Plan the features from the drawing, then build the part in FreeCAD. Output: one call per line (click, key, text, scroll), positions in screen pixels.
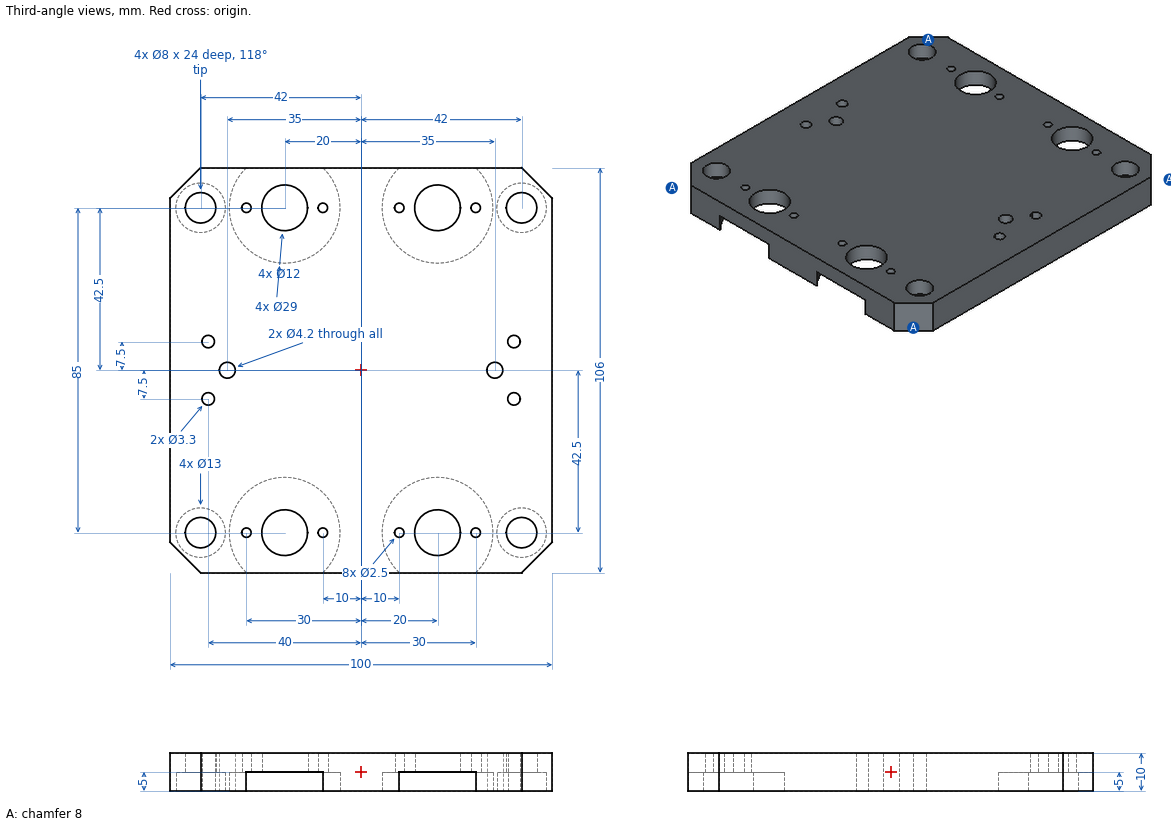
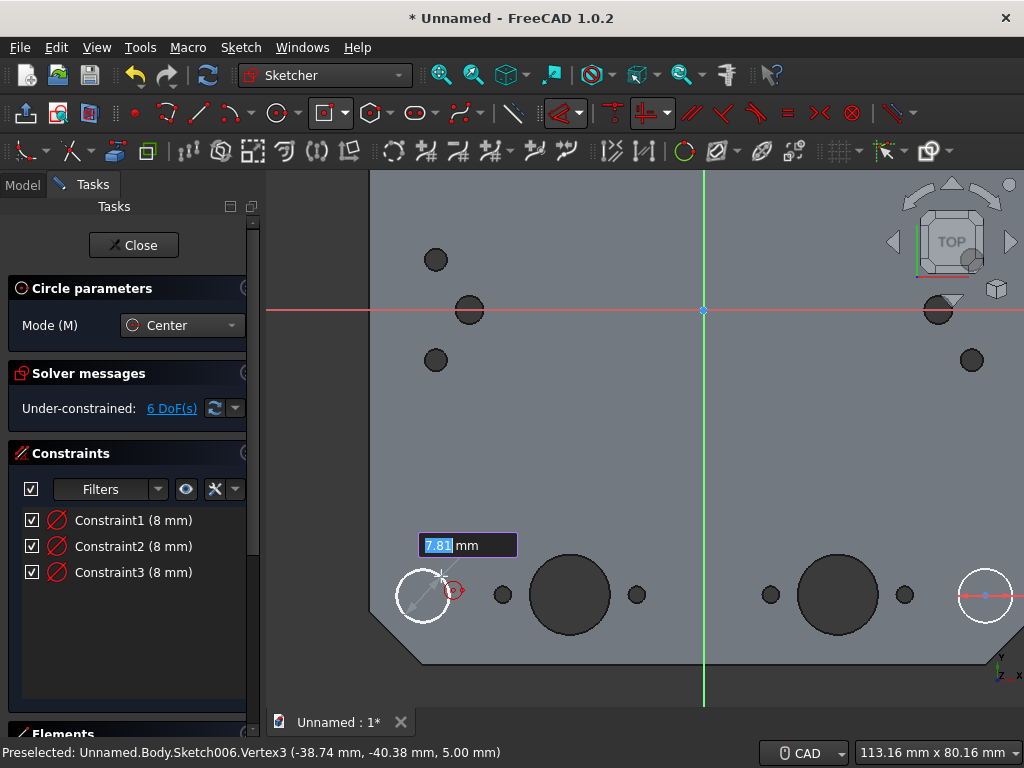
text(8)
key(Return)
key(Escape)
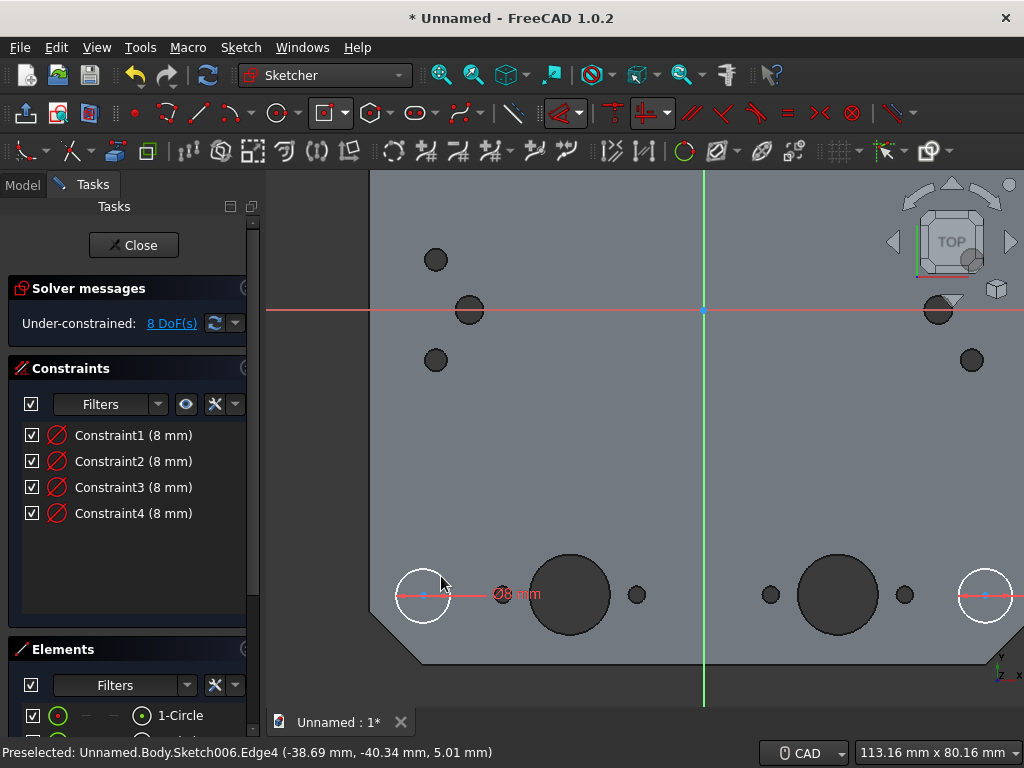
scroll(422, 595, down, 3)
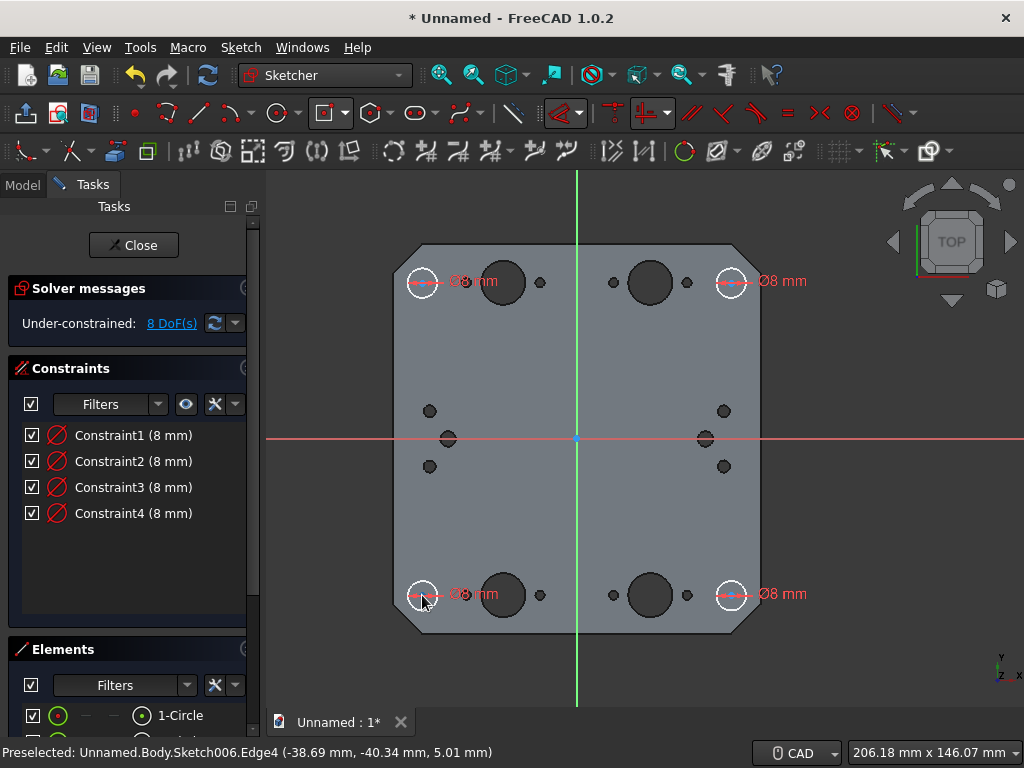
click(422, 283)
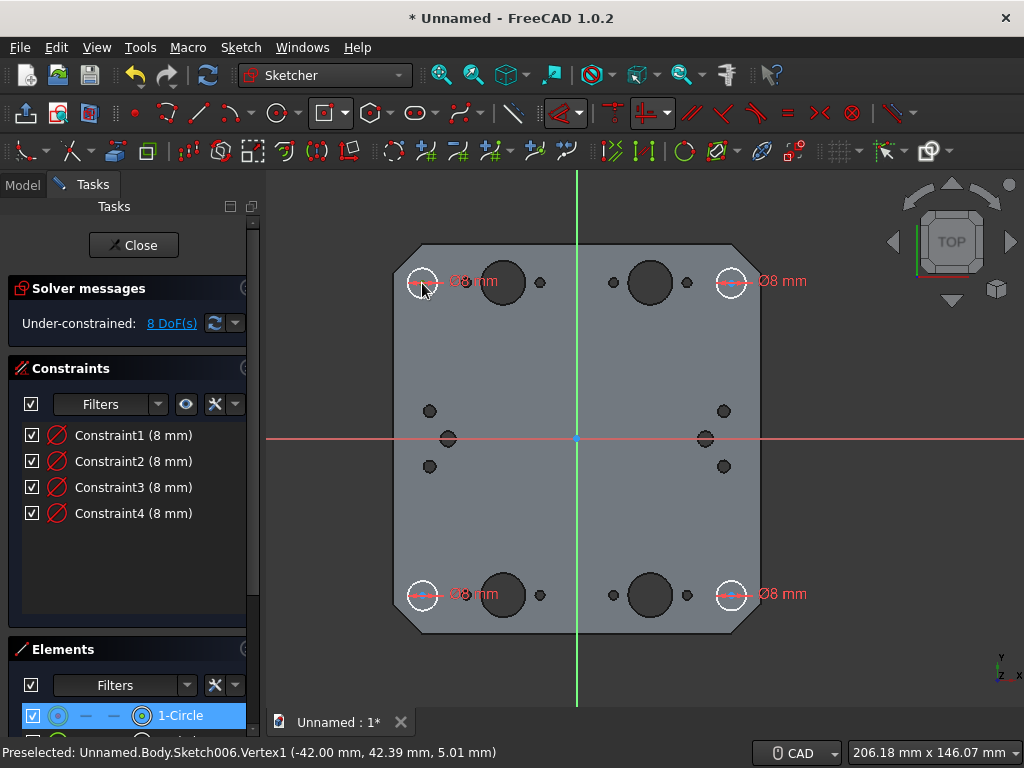
click(731, 283)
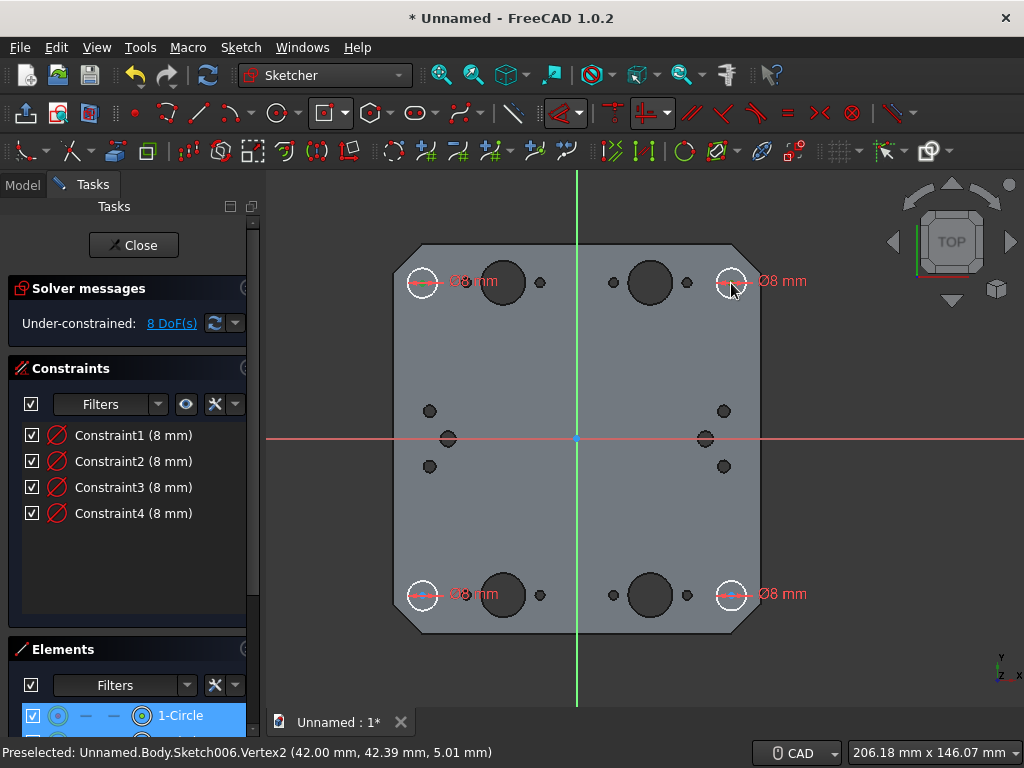
click(670, 114)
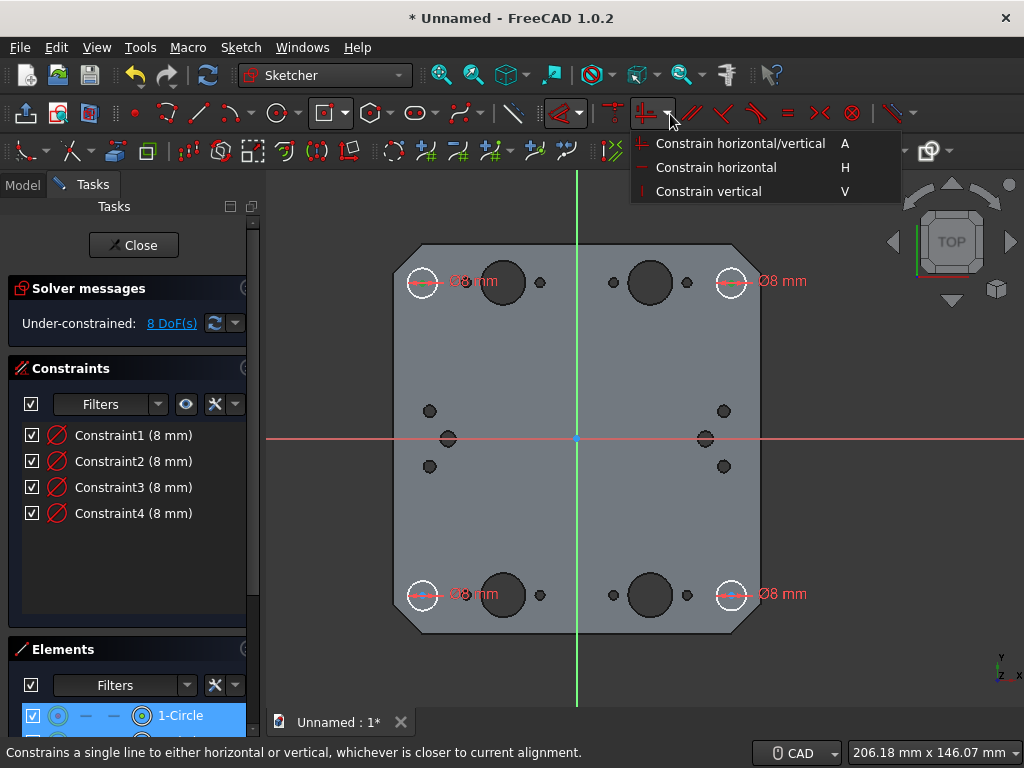
click(766, 167)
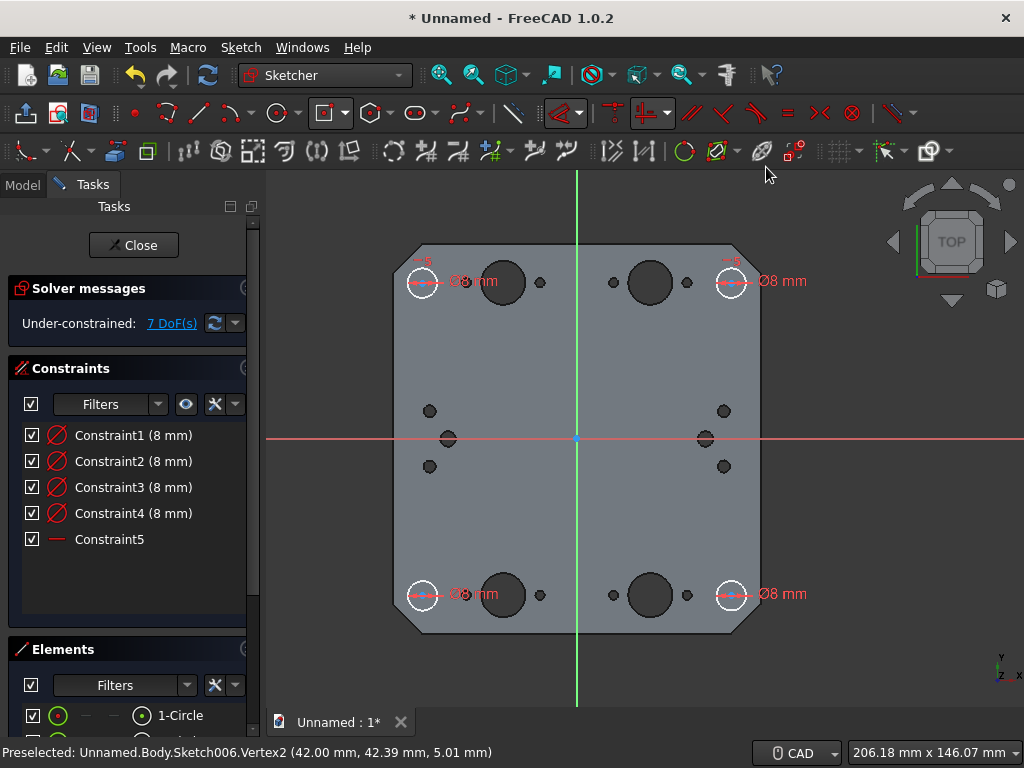
click(731, 283)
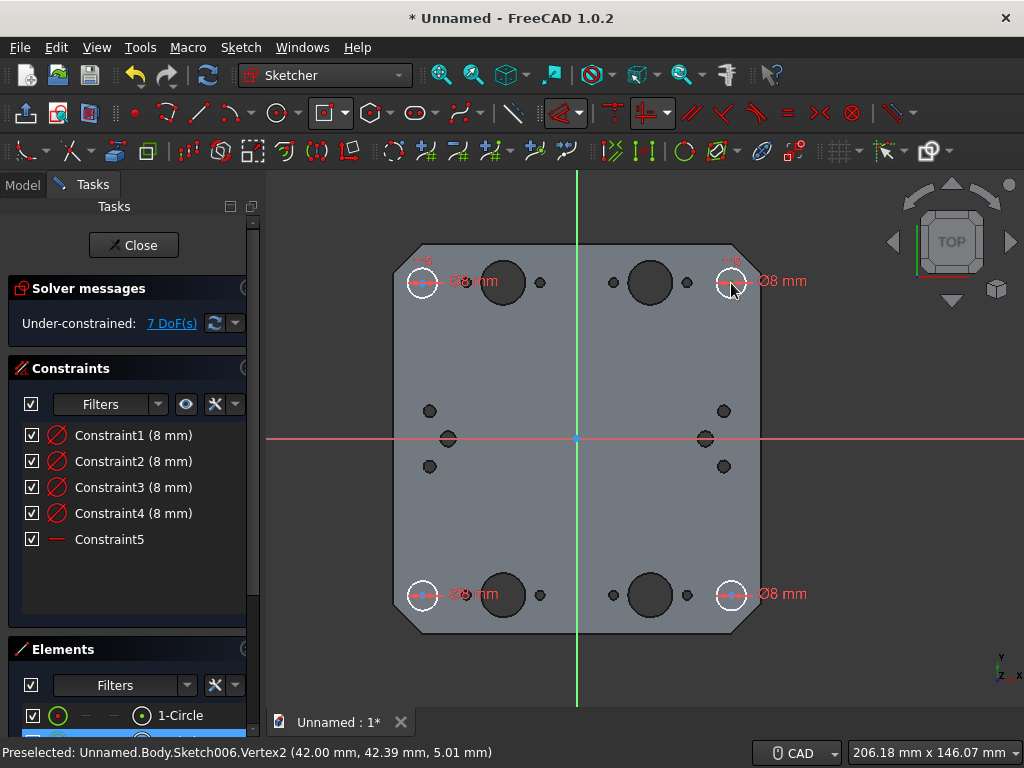
click(731, 596)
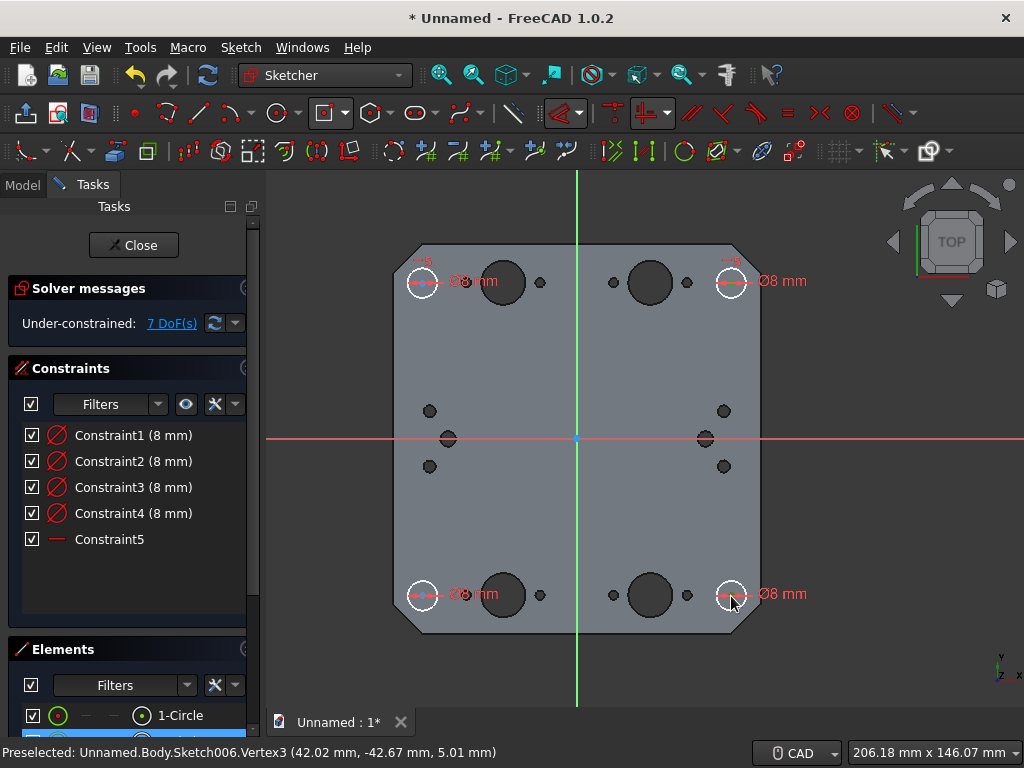
click(670, 114)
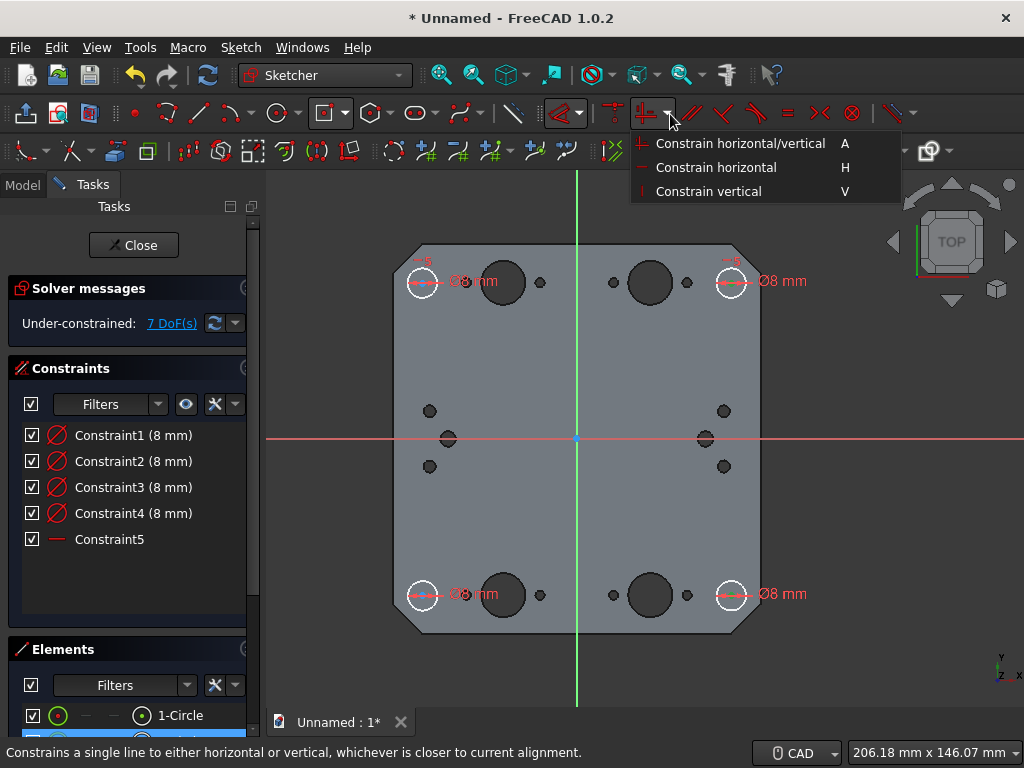
click(766, 191)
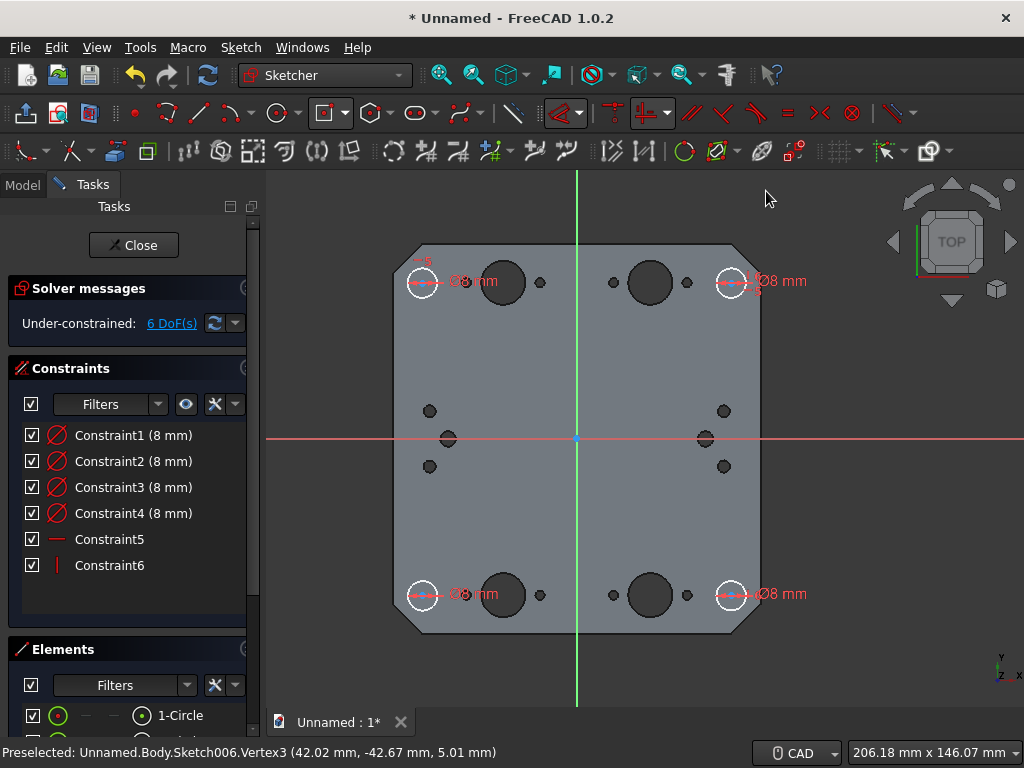
click(422, 283)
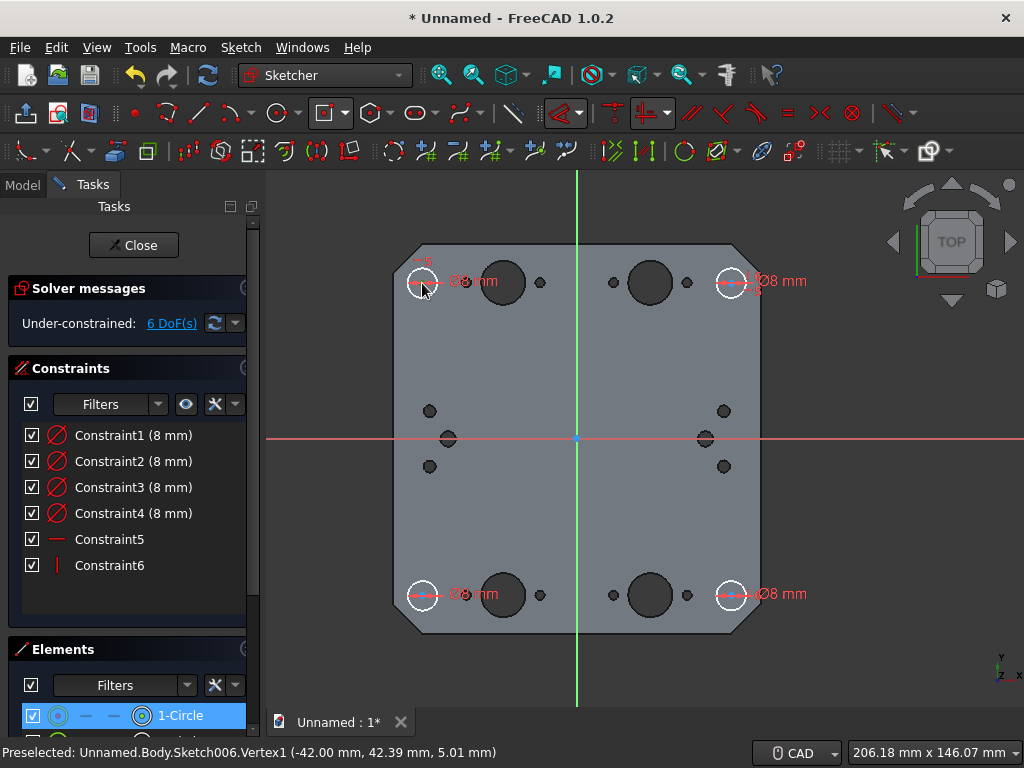
click(423, 596)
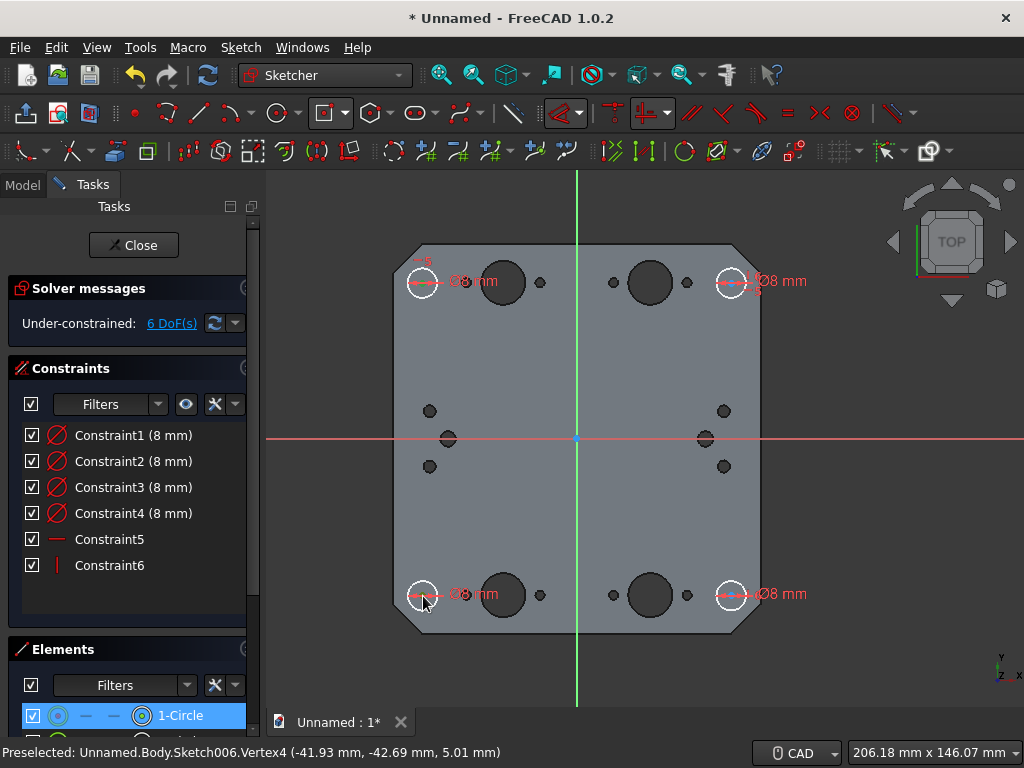
key(v)